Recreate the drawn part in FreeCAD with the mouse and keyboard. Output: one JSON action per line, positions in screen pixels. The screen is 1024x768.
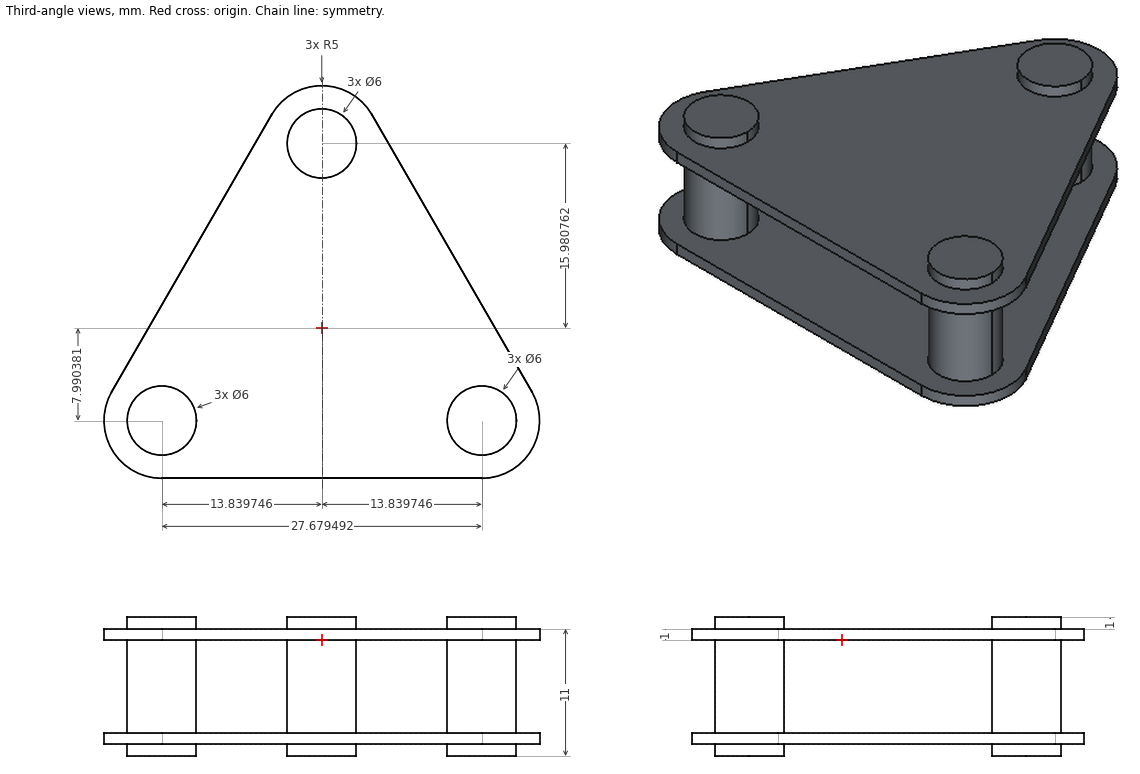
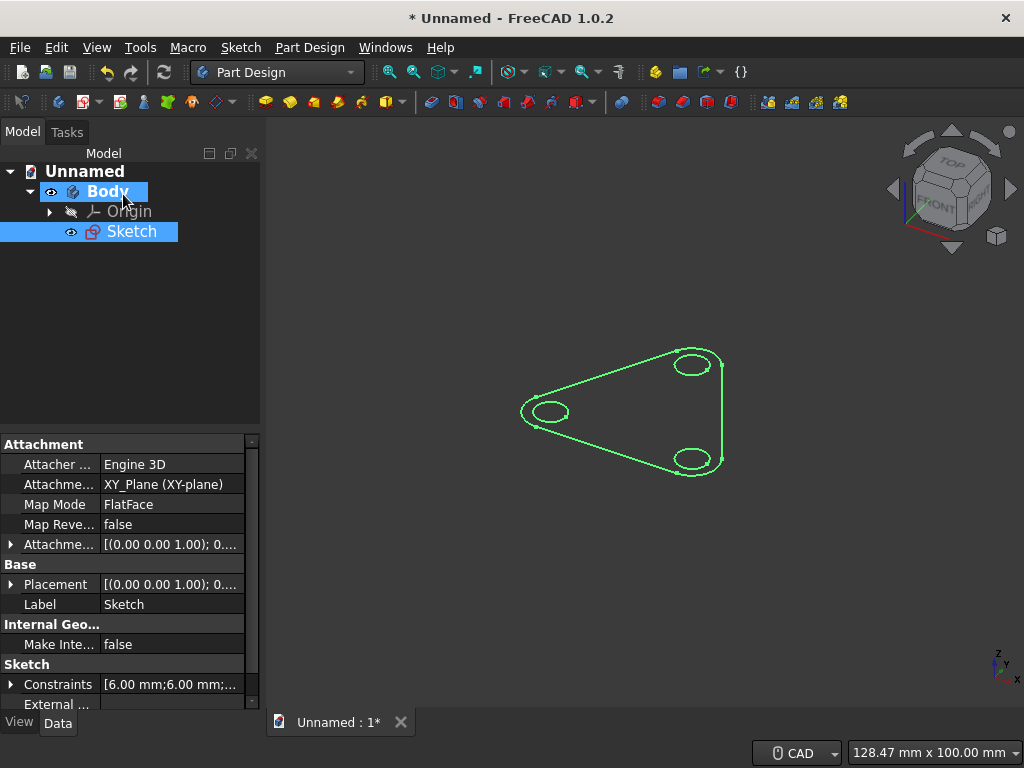
{"action": "left_click", "coordinate": [266, 102]}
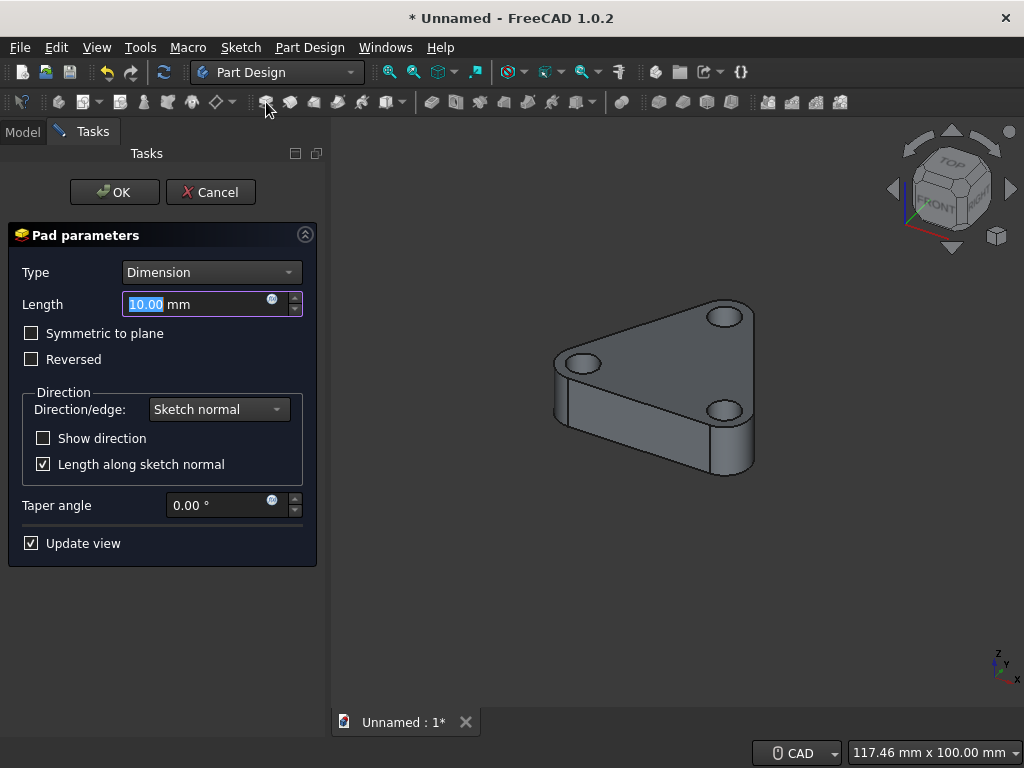
{"action": "type", "text": "1"}
{"action": "key", "text": "Tab"}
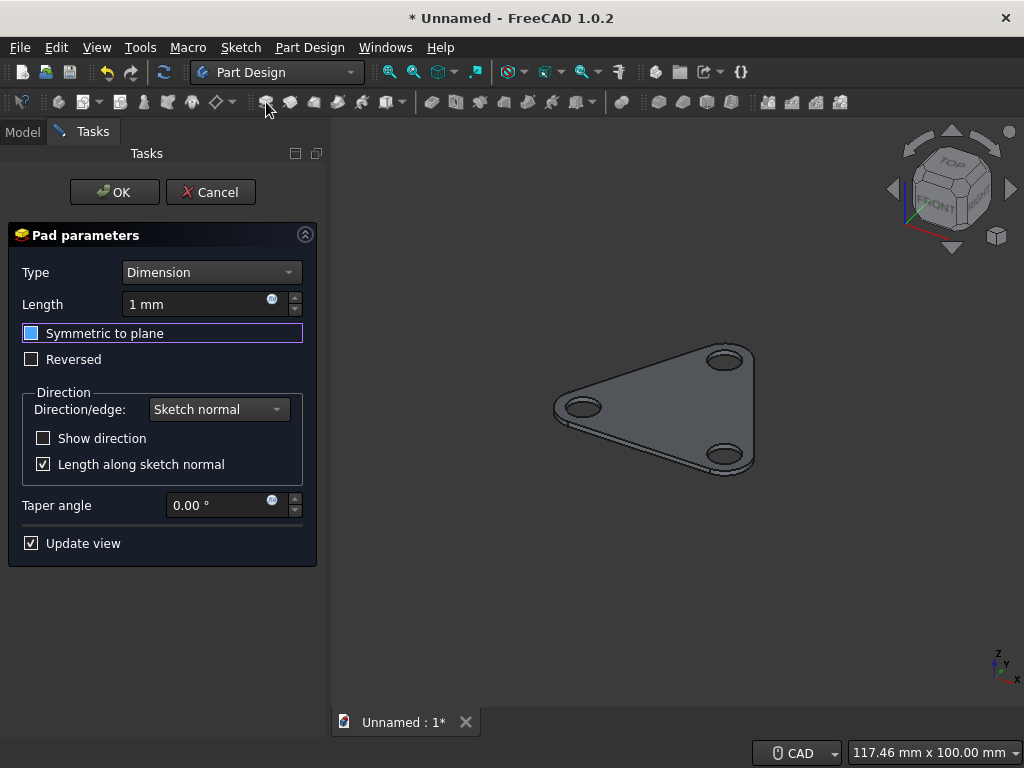
{"action": "left_click", "coordinate": [115, 192]}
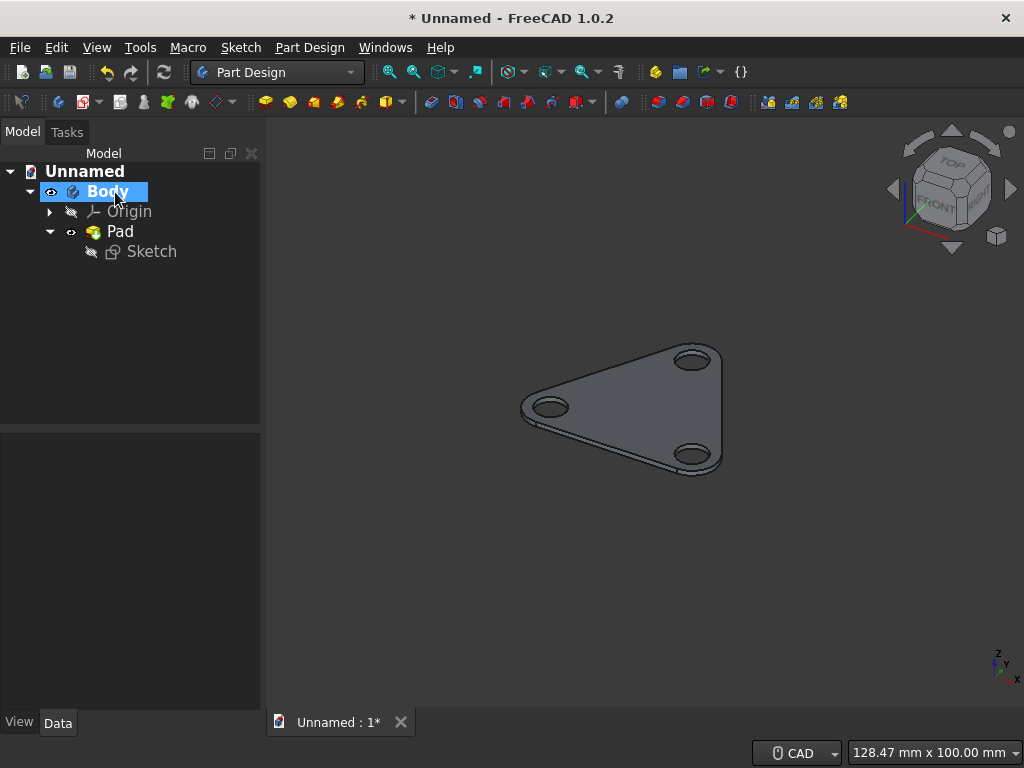
{"action": "left_click", "coordinate": [390, 72]}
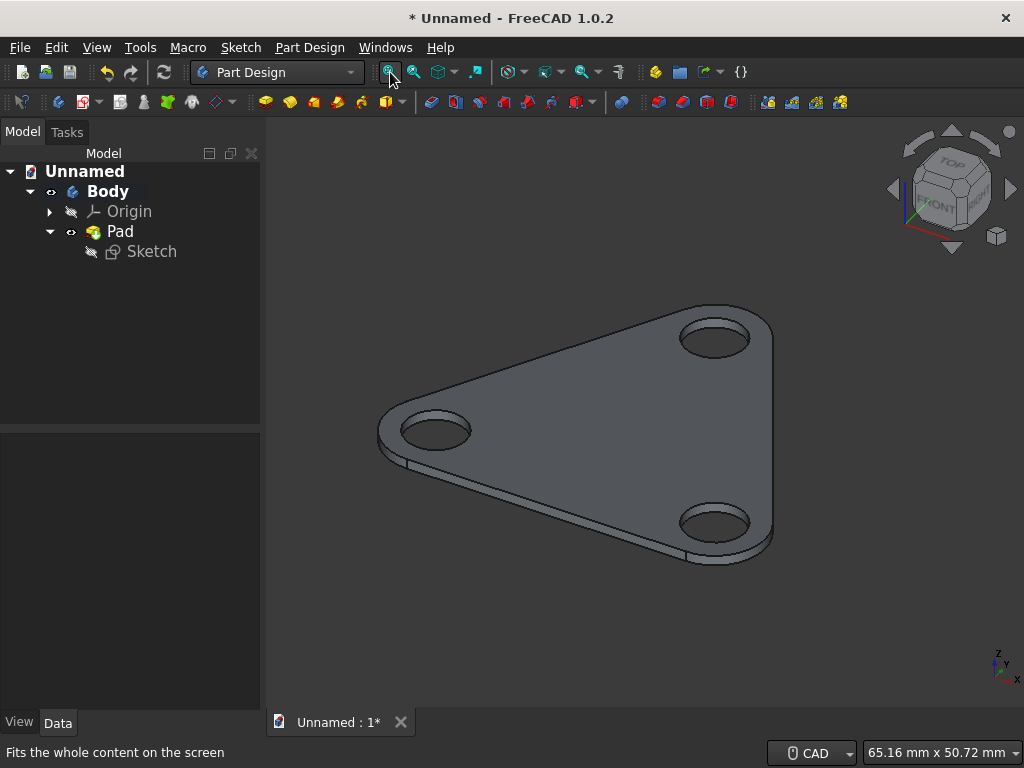
{"action": "left_click", "coordinate": [50, 212]}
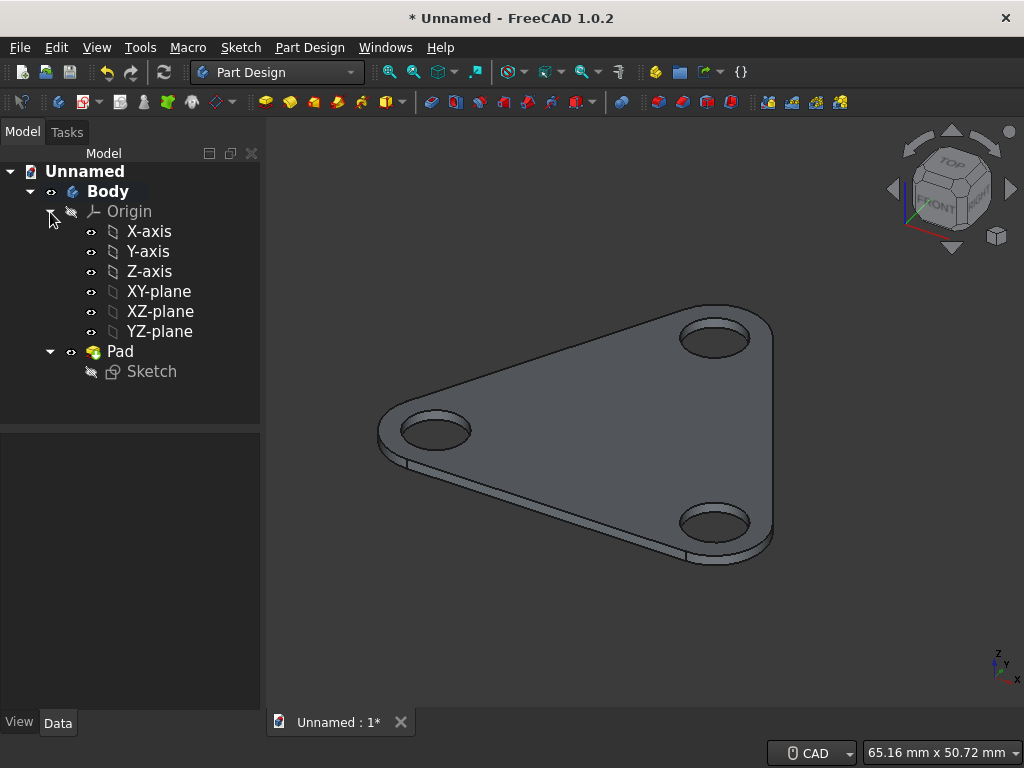
{"action": "left_click", "coordinate": [136, 292]}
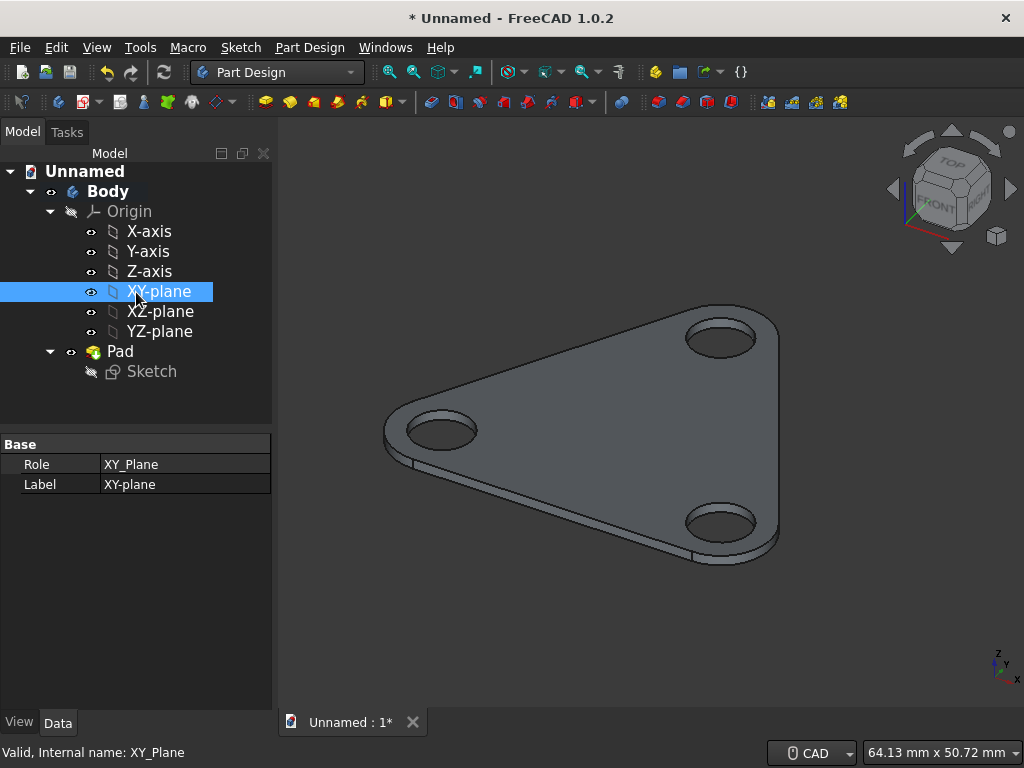
{"action": "left_click", "coordinate": [216, 102]}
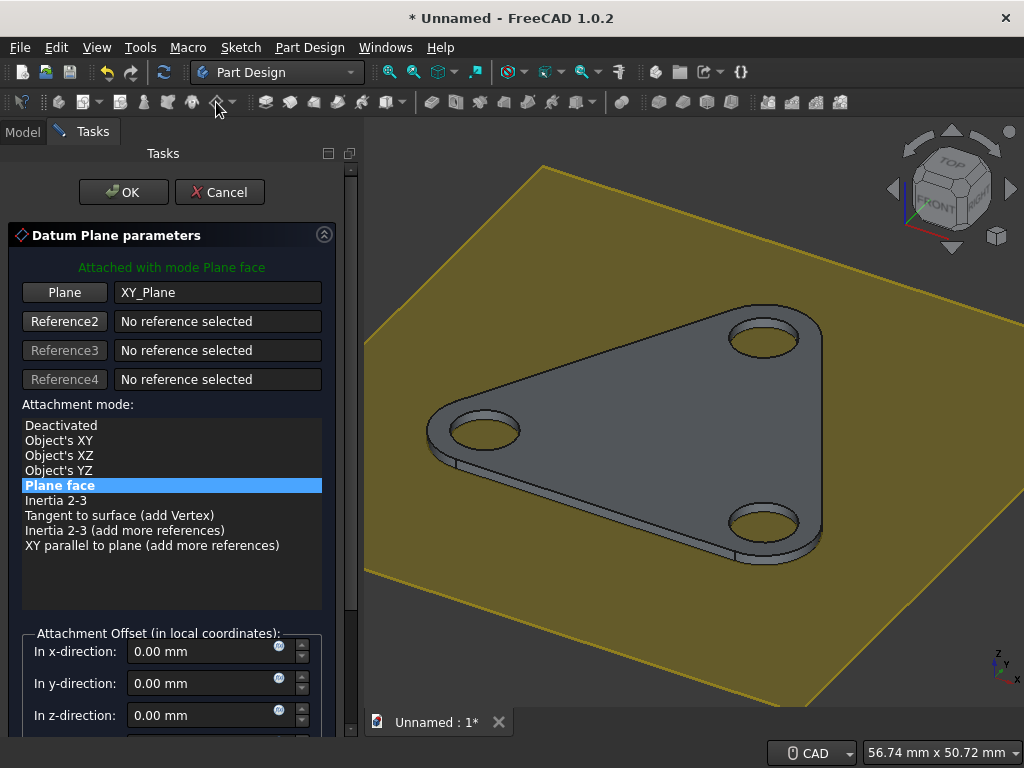
{"action": "triple_click", "coordinate": [210, 715]}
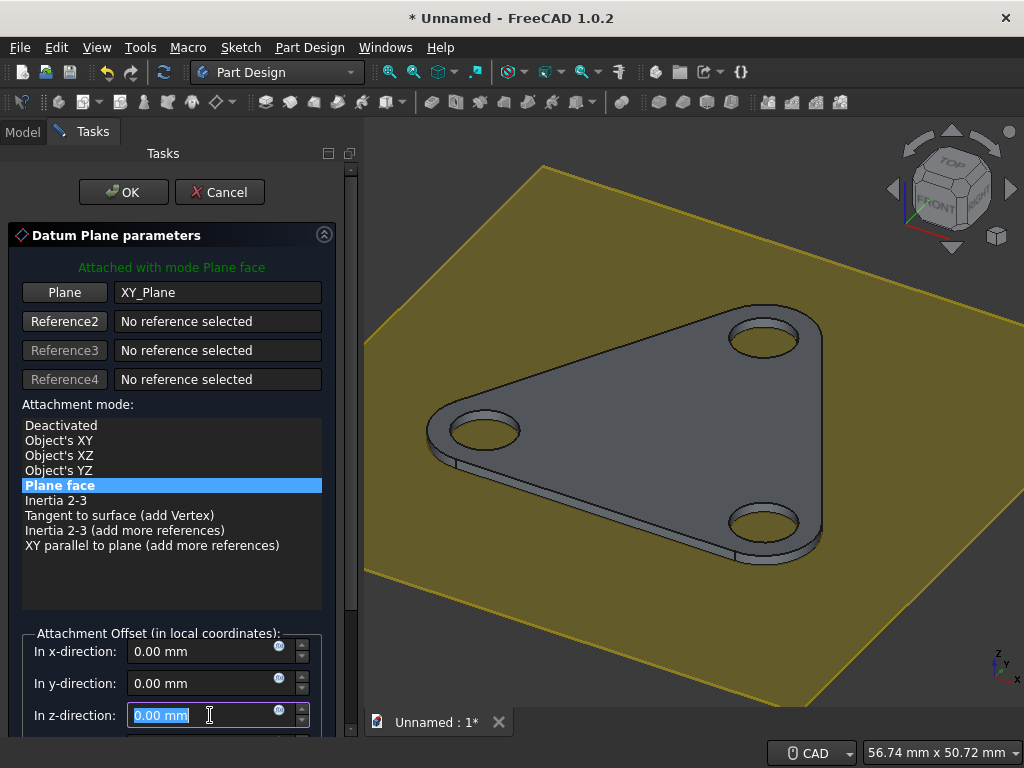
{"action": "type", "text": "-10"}
{"action": "key", "text": "Tab"}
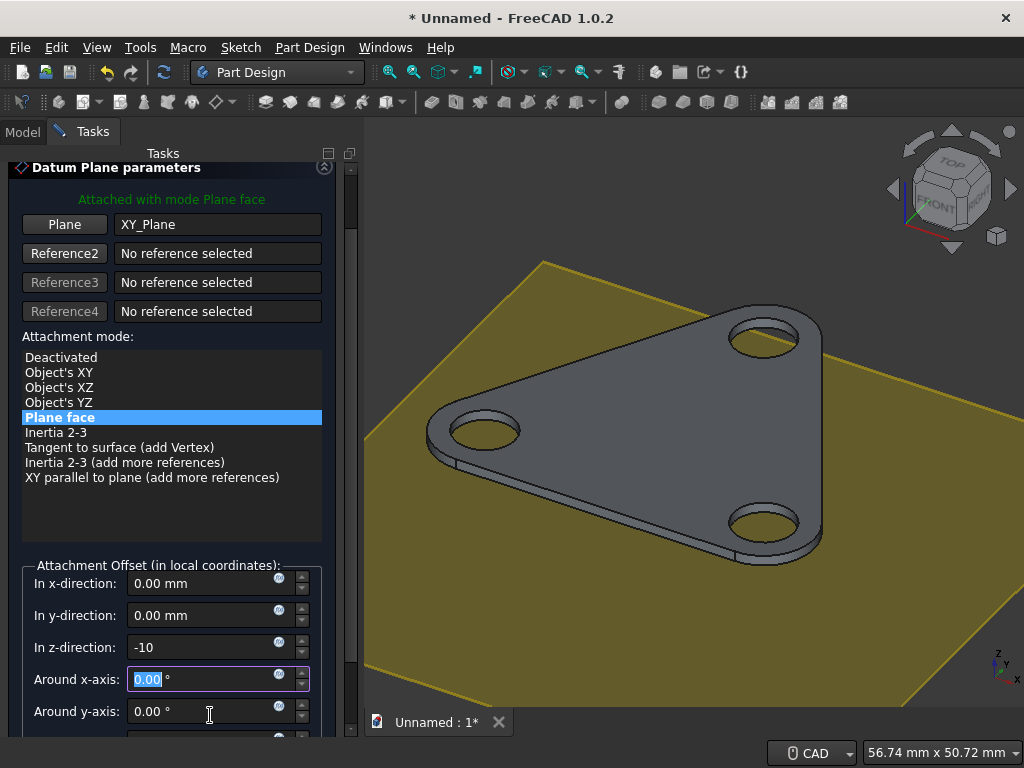
{"action": "scroll", "coordinate": [351, 450], "scroll_direction": "up", "scroll_amount": 2}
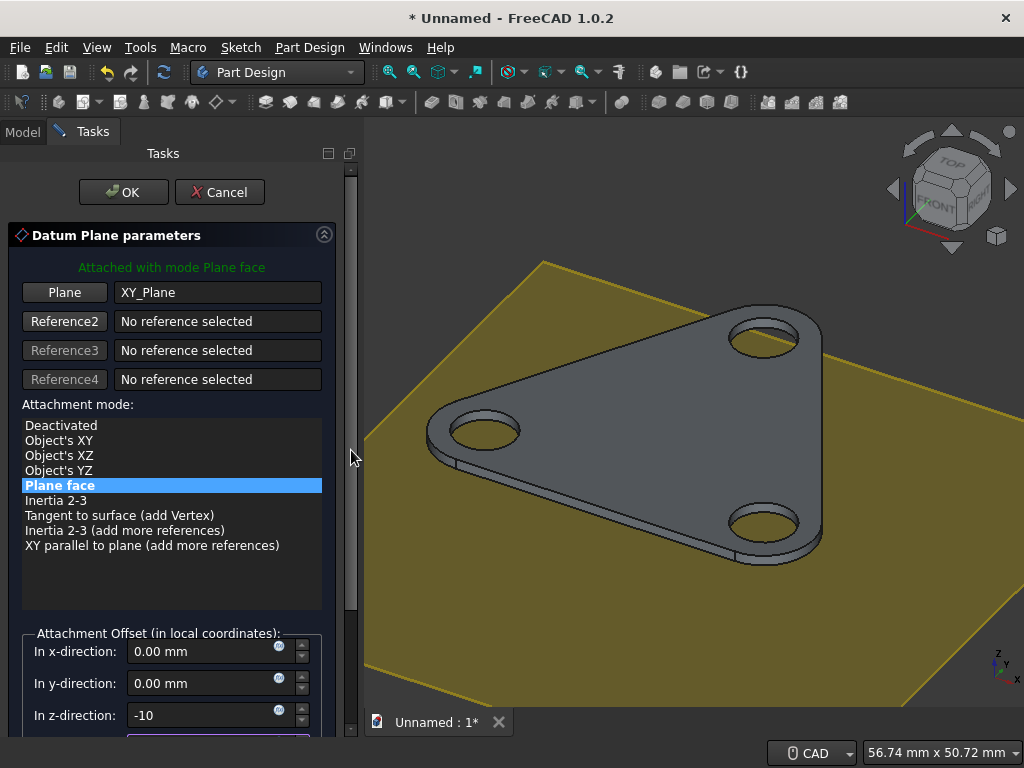
{"action": "left_click", "coordinate": [124, 192]}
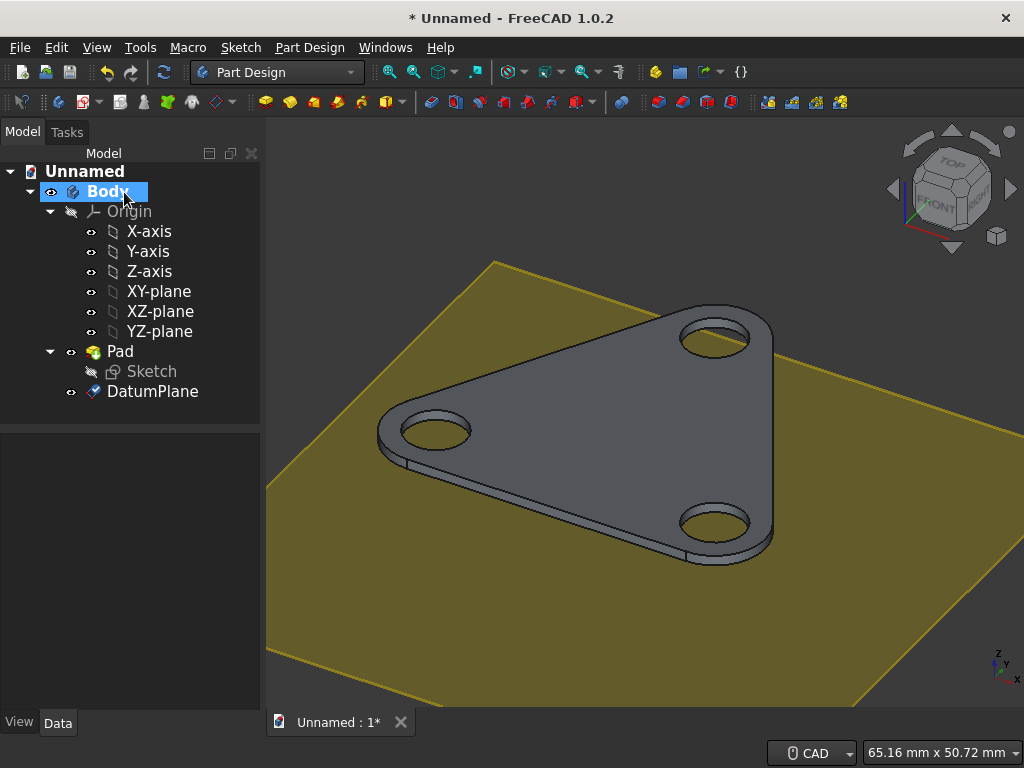
{"action": "left_click", "coordinate": [116, 392]}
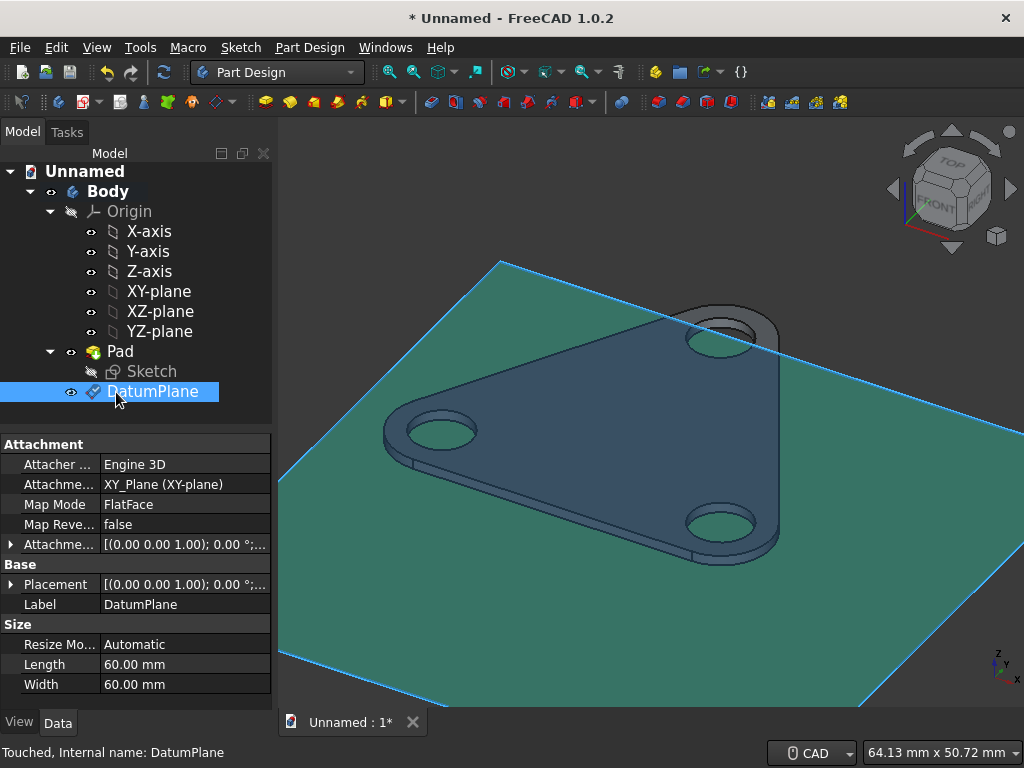
{"action": "left_click", "coordinate": [84, 102]}